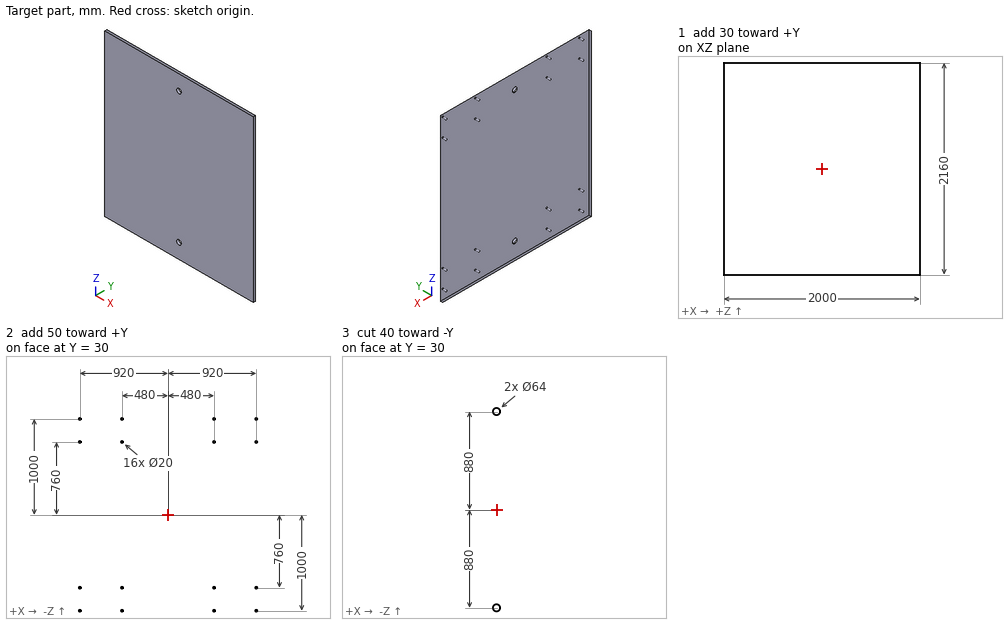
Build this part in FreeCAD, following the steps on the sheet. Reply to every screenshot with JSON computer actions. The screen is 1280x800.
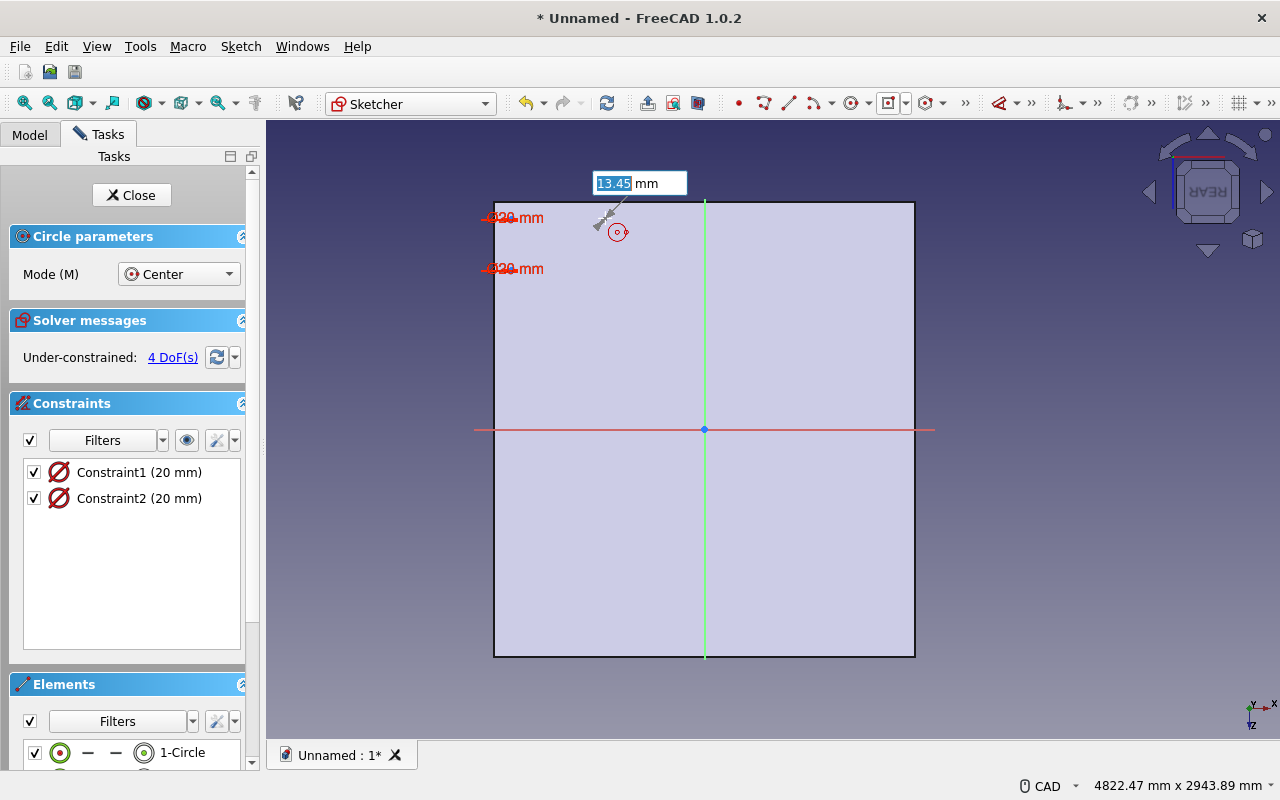
{"action": "type", "text": "20"}
{"action": "key", "text": "Return"}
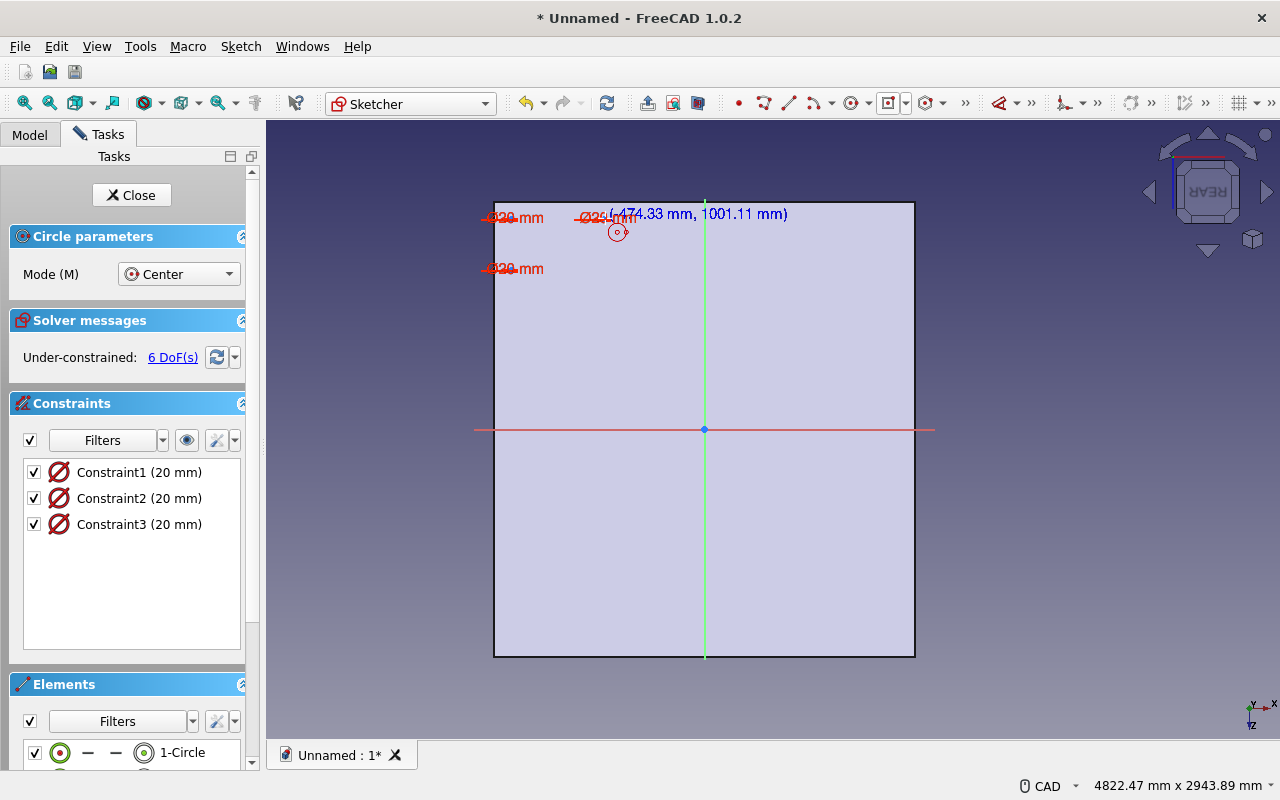
{"action": "scroll", "coordinate": [604, 270], "scroll_direction": "up", "scroll_amount": 12}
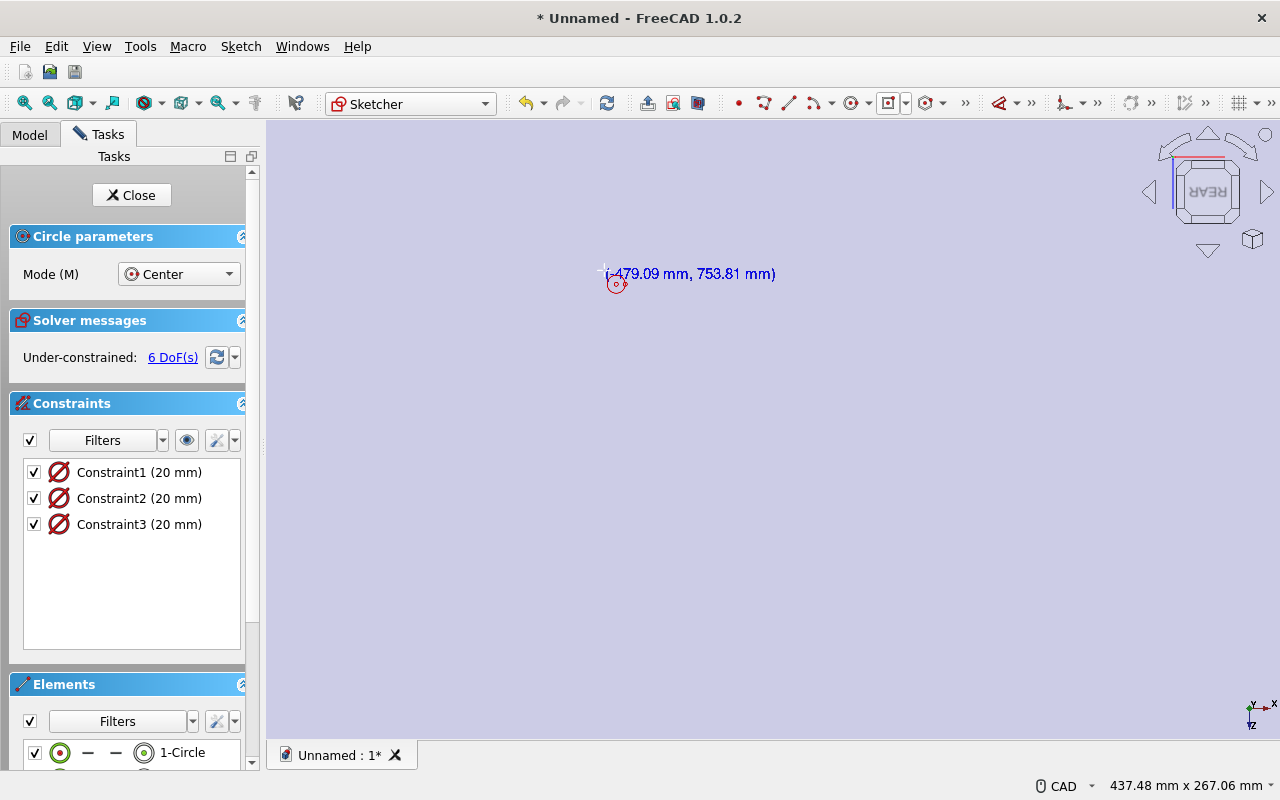
{"action": "scroll", "coordinate": [604, 270], "scroll_direction": "down", "scroll_amount": 12}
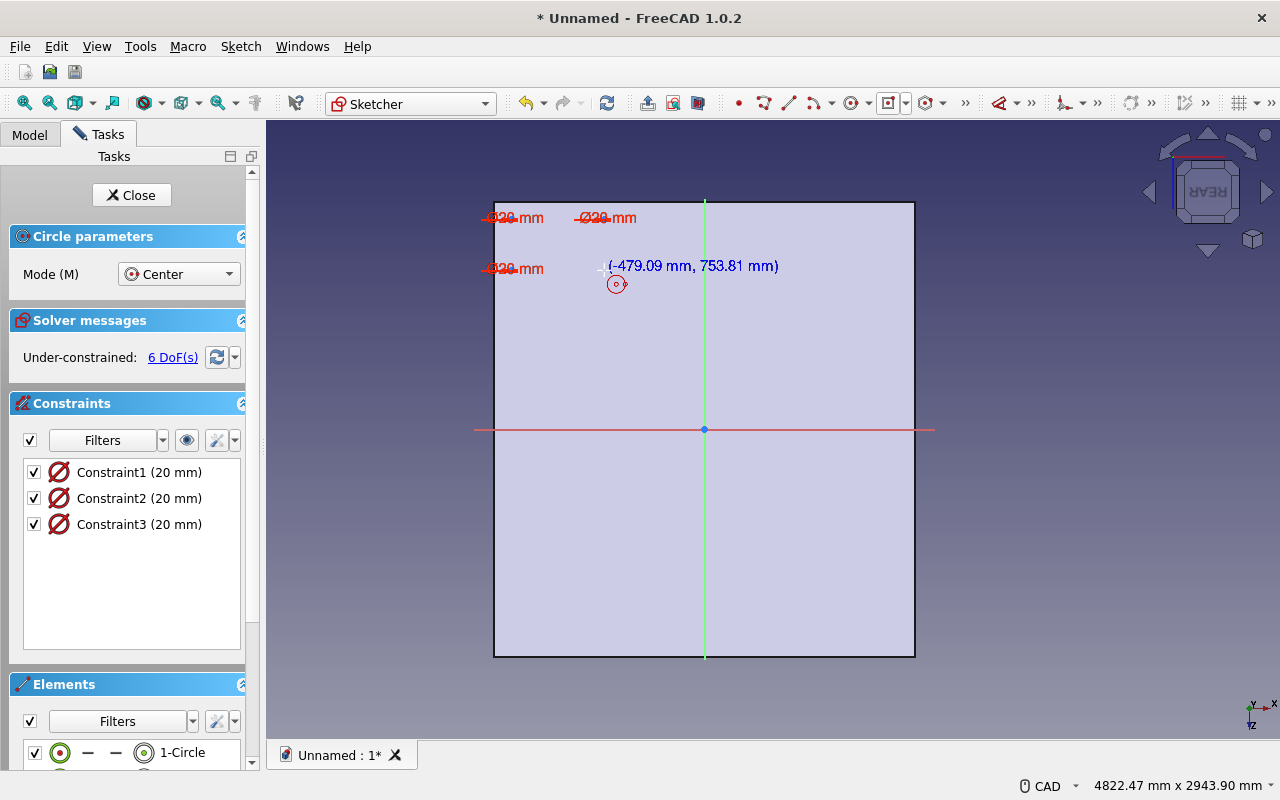
{"action": "left_click", "coordinate": [604, 270]}
{"action": "mouse_move", "coordinate": [605, 268]}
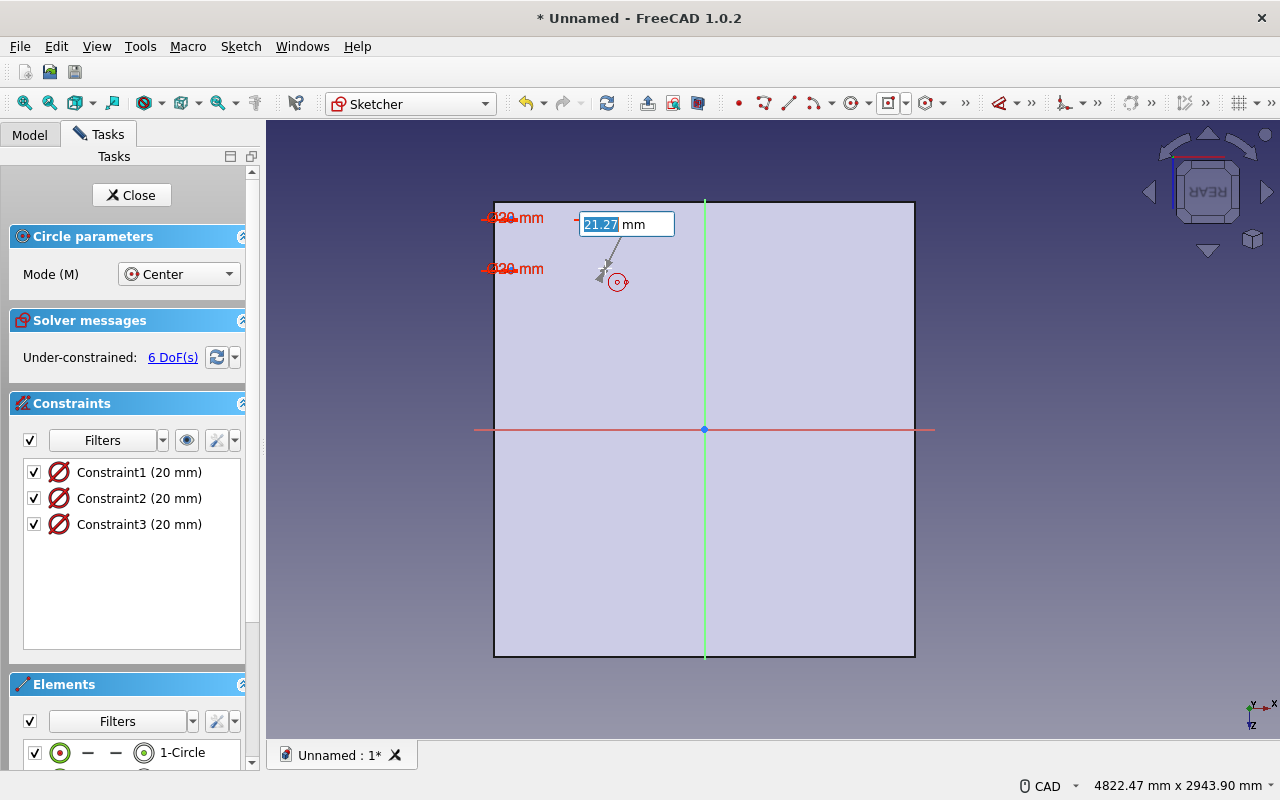
{"action": "type", "text": "20"}
{"action": "key", "text": "Return"}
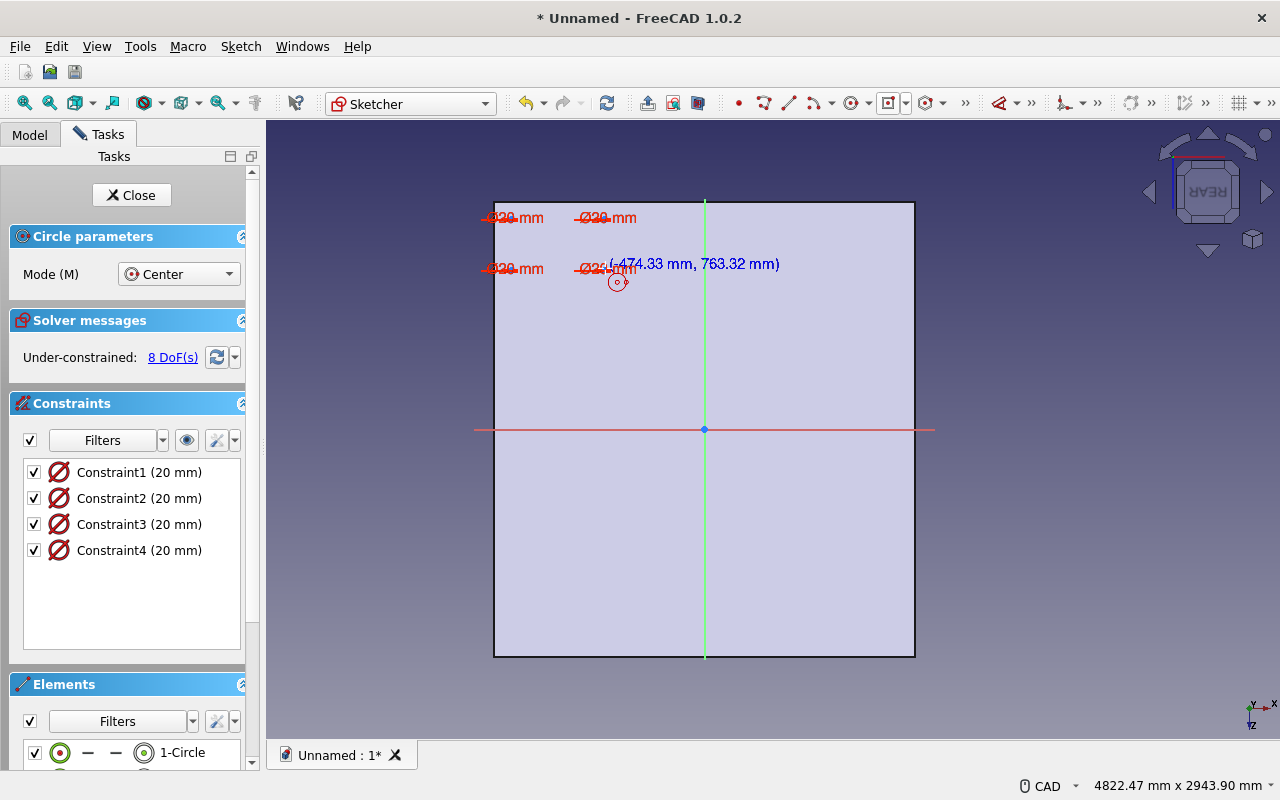
{"action": "scroll", "coordinate": [806, 270], "scroll_direction": "up", "scroll_amount": 12}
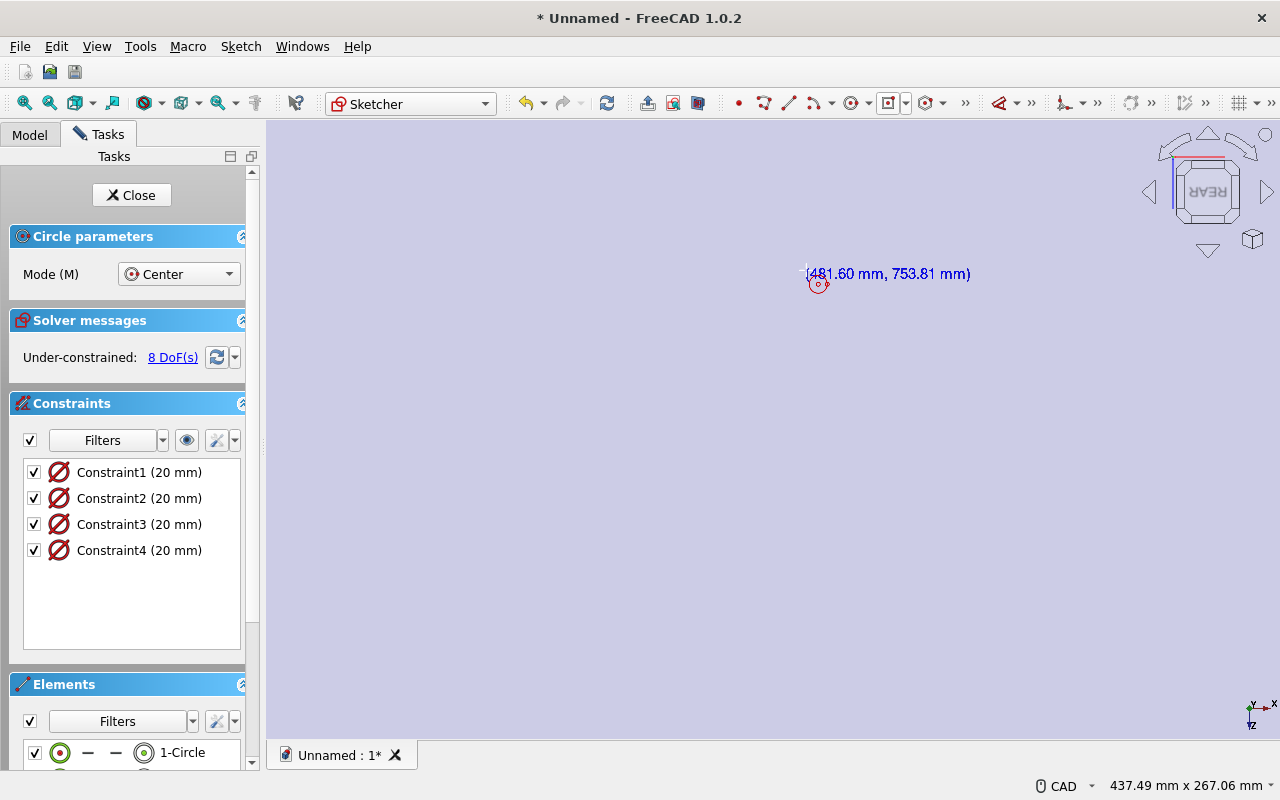
{"action": "scroll", "coordinate": [806, 270], "scroll_direction": "down", "scroll_amount": 12}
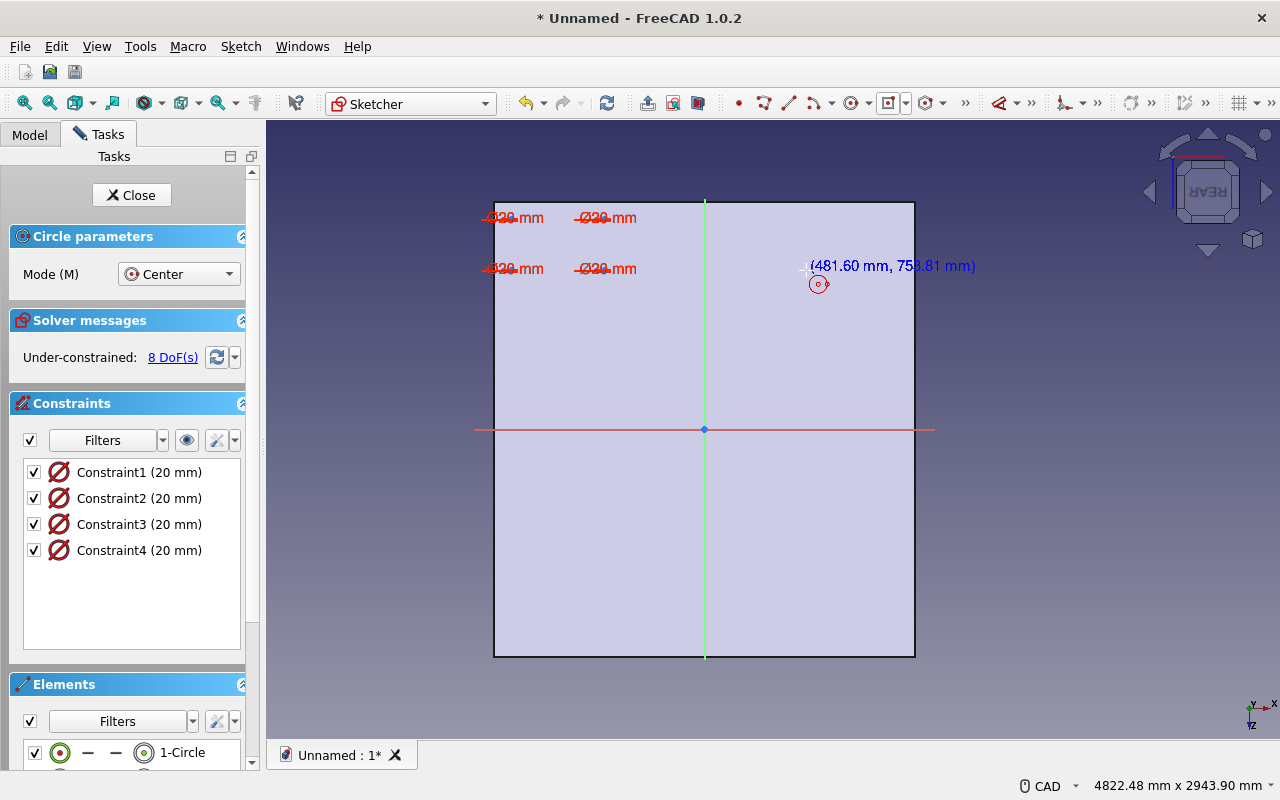
{"action": "left_click", "coordinate": [806, 270]}
{"action": "mouse_move", "coordinate": [807, 268]}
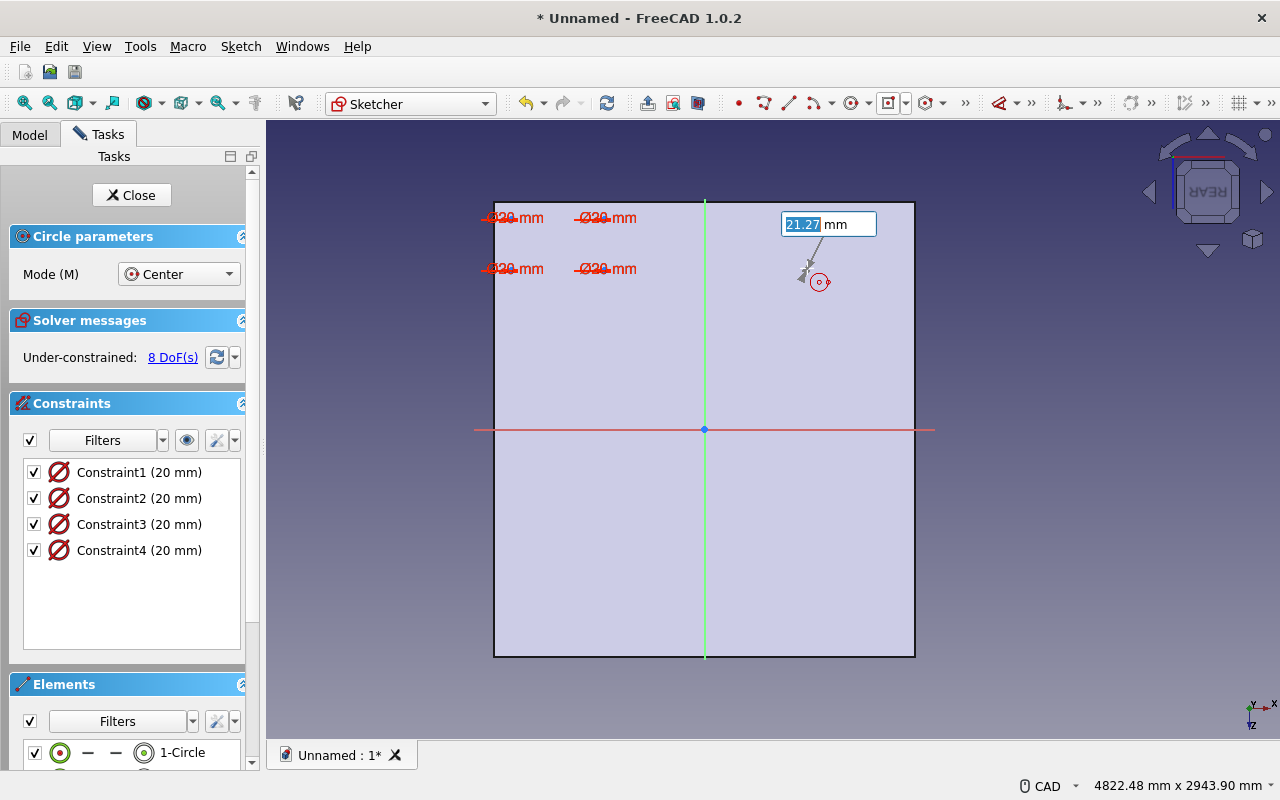
{"action": "type", "text": "20"}
{"action": "key", "text": "Return"}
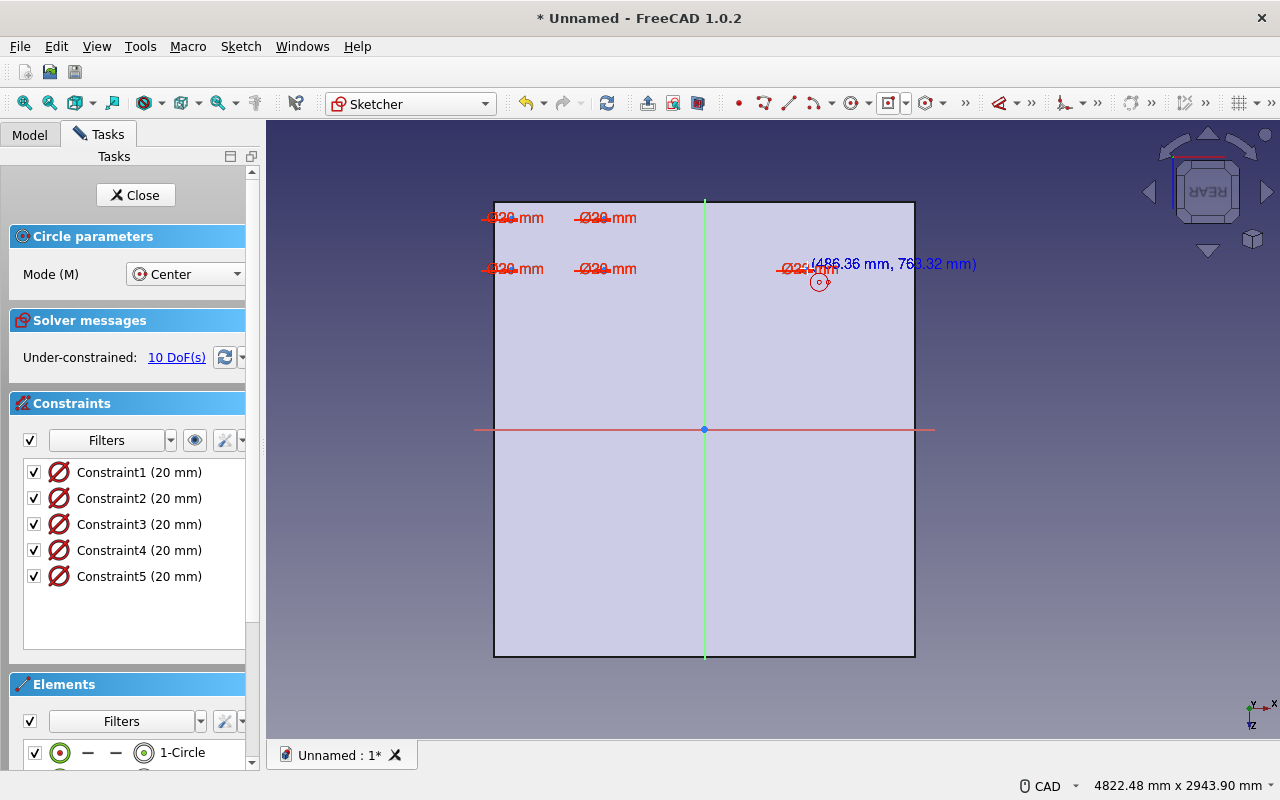
{"action": "scroll", "coordinate": [806, 219], "scroll_direction": "up", "scroll_amount": 12}